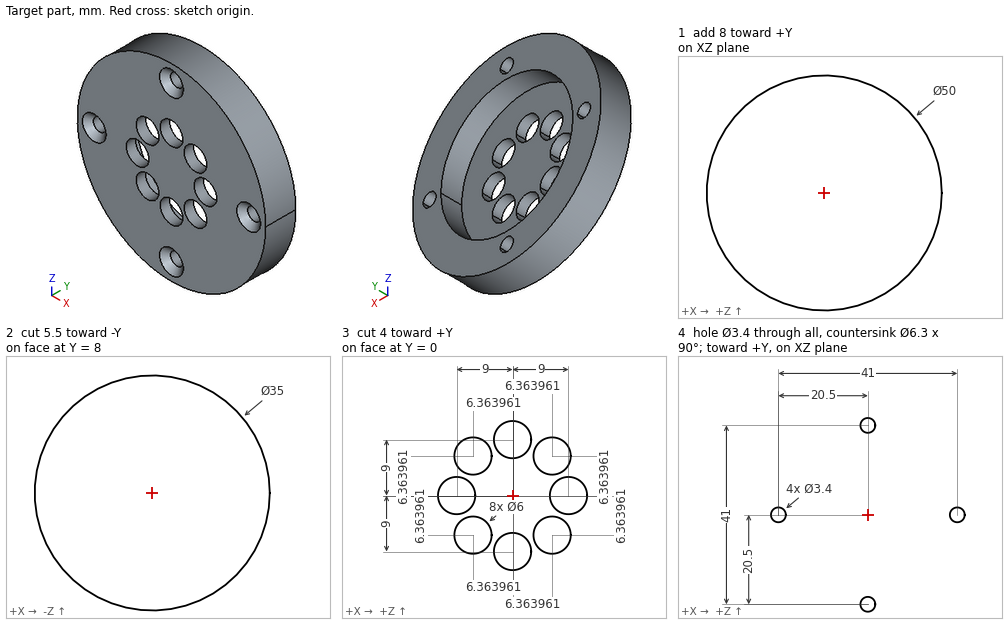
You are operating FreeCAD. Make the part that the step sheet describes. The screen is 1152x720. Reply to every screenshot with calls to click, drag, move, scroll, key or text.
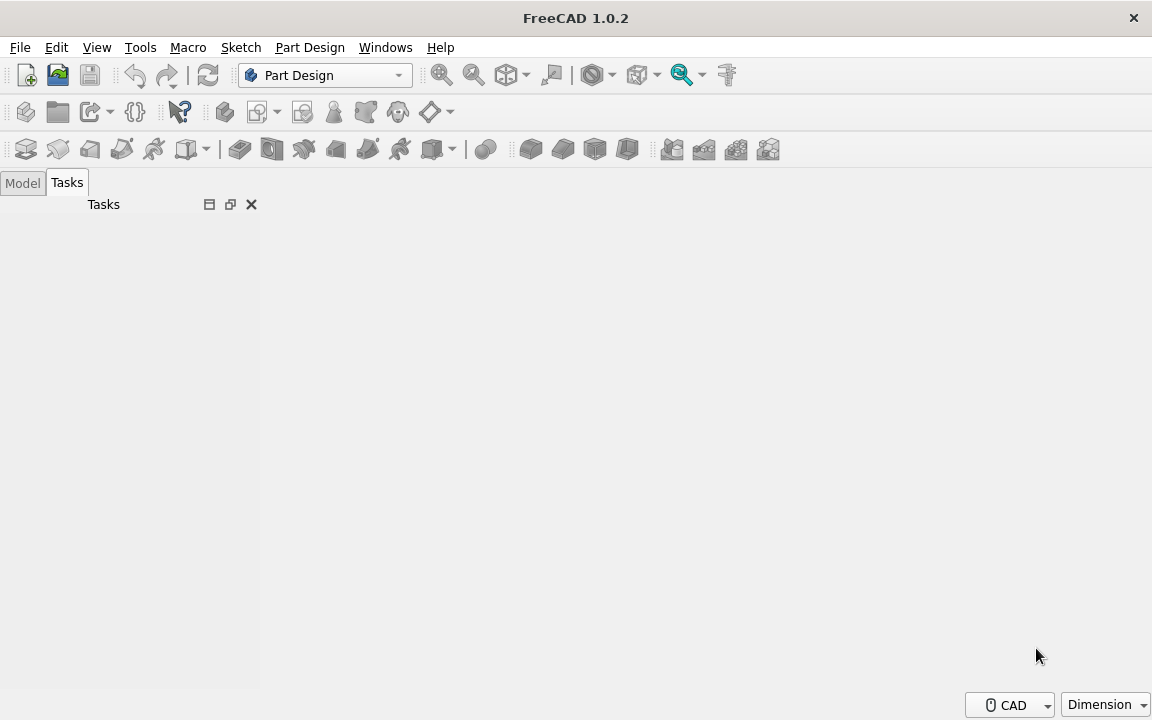
click(26, 76)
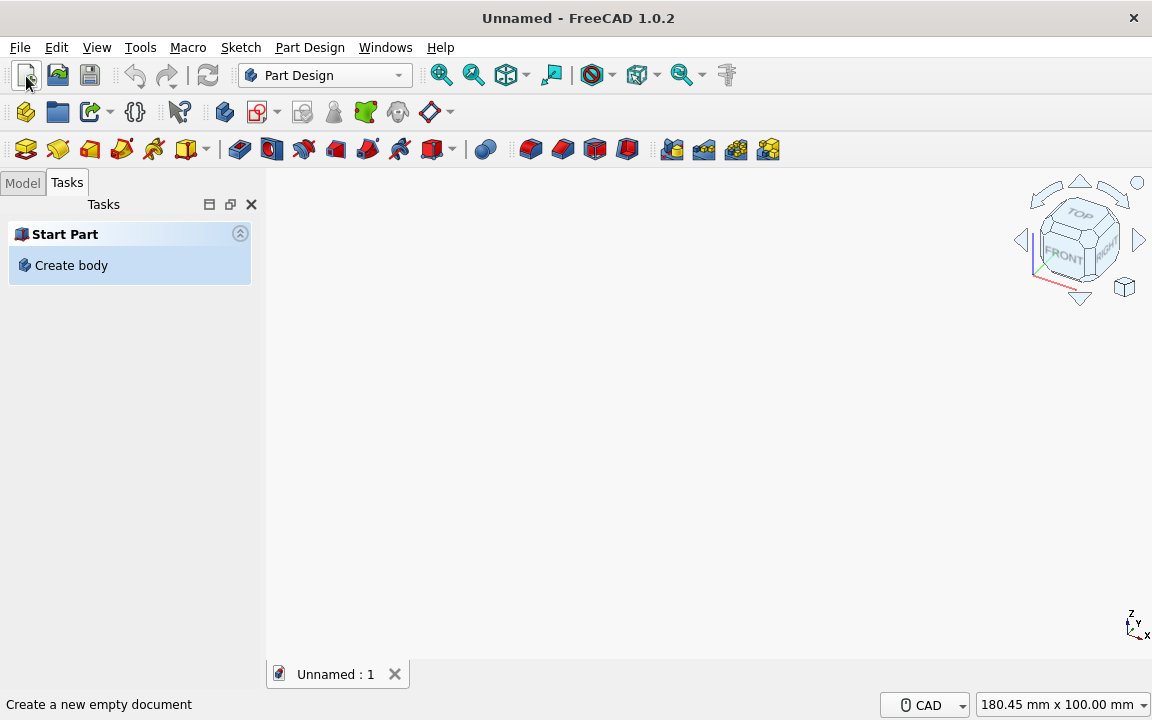
click(258, 112)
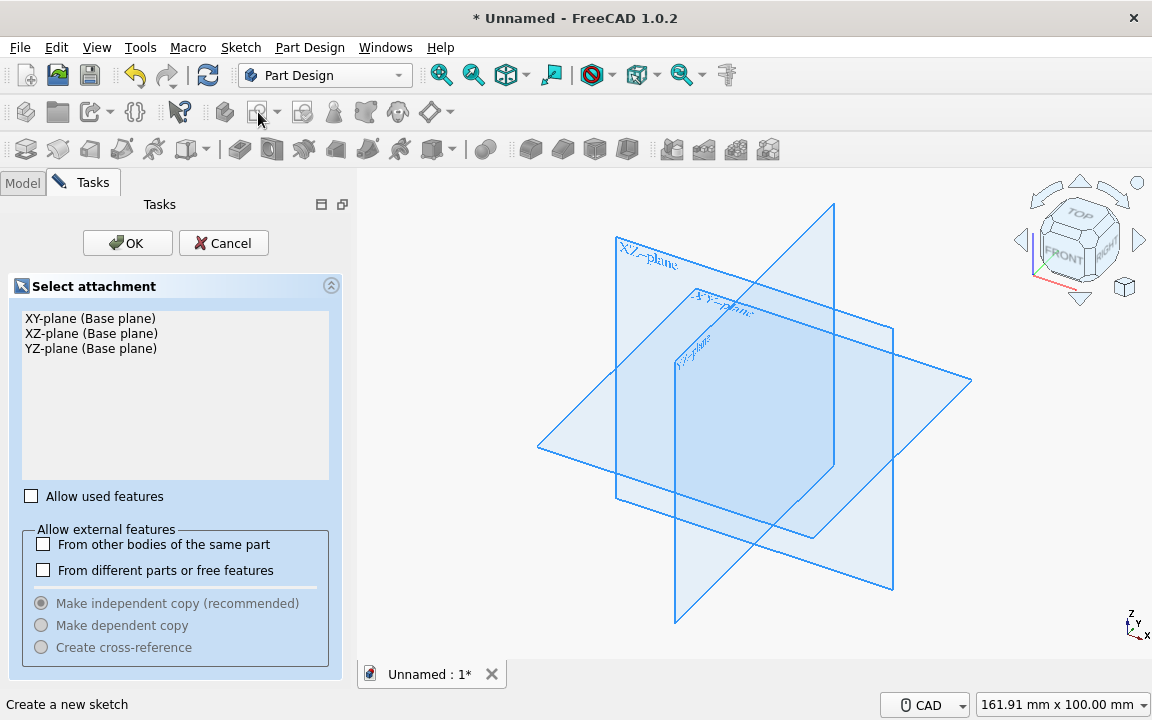
click(82, 334)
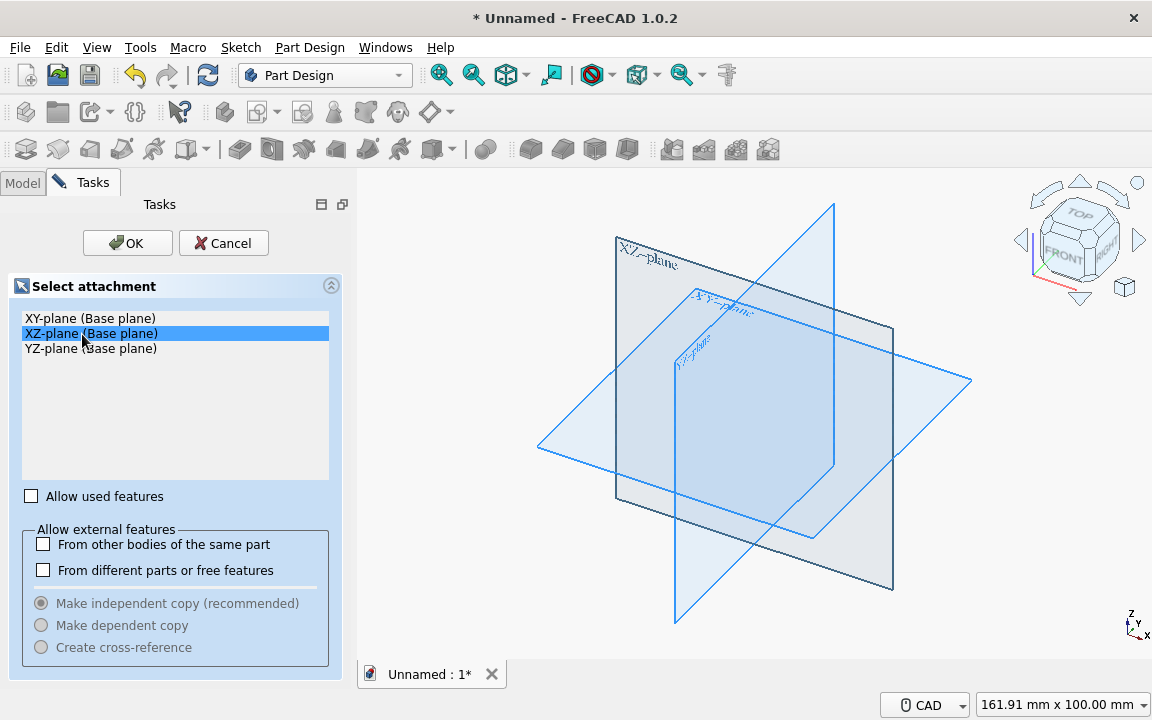
click(128, 243)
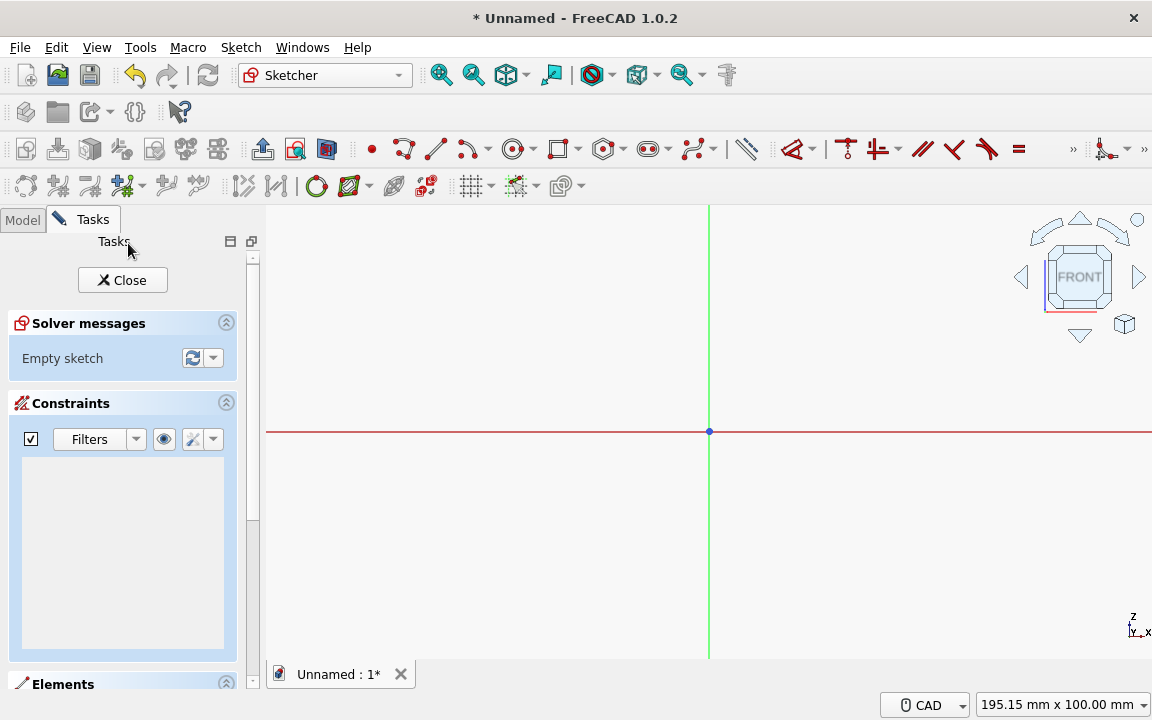
key(g)
key(c)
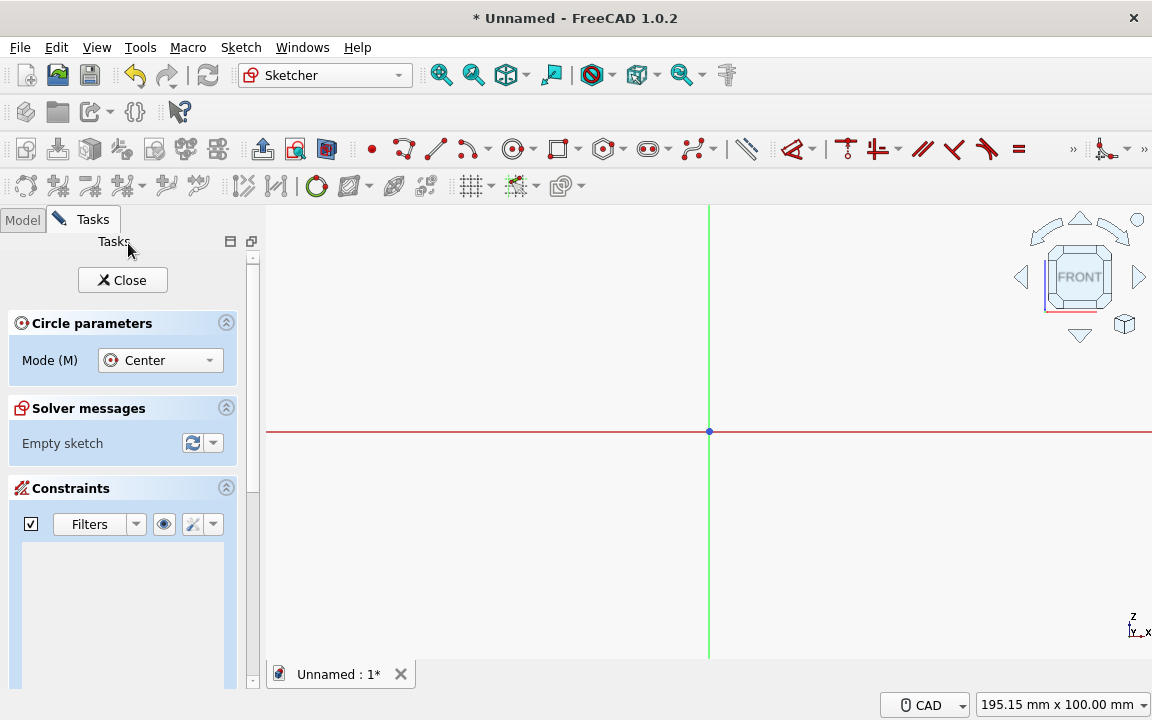
click(709, 432)
move(789, 352)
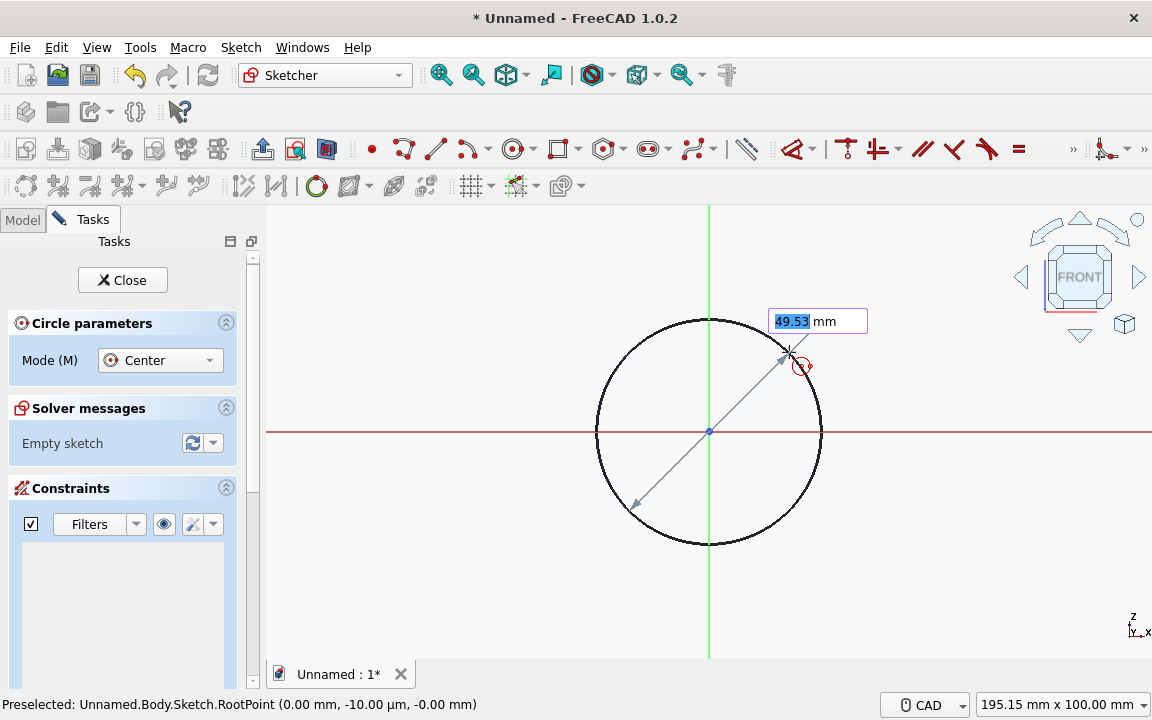
text(50)
key(Return)
key(Escape)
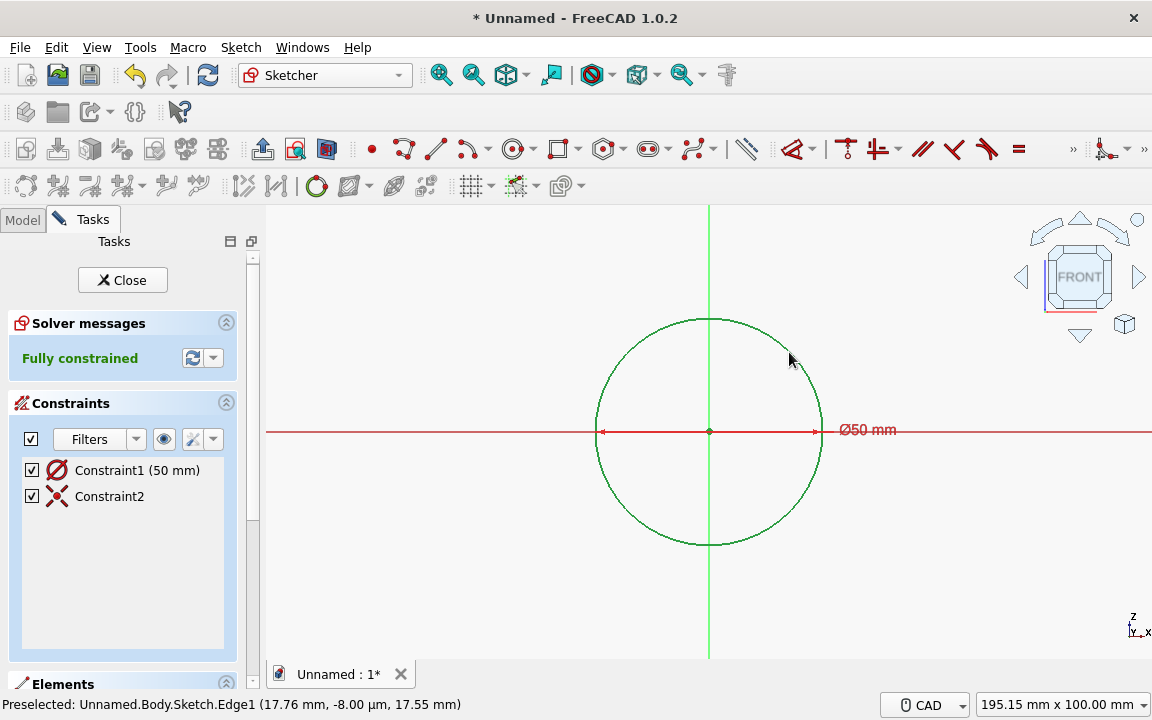
click(123, 280)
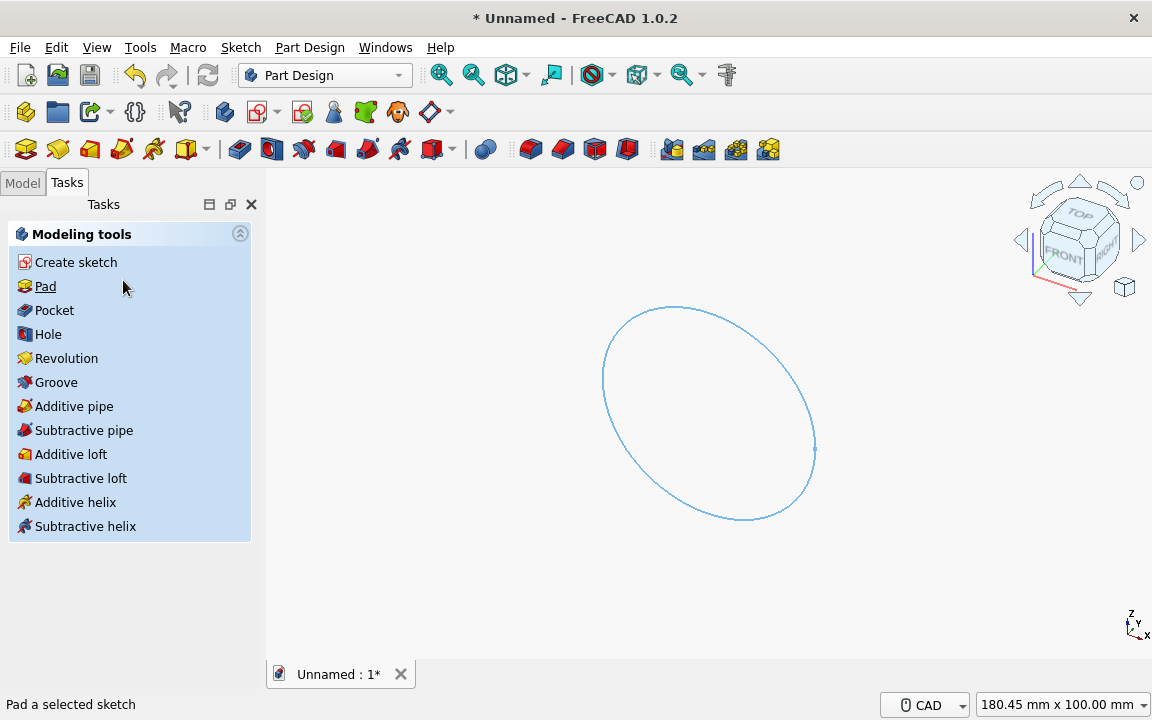
click(26, 150)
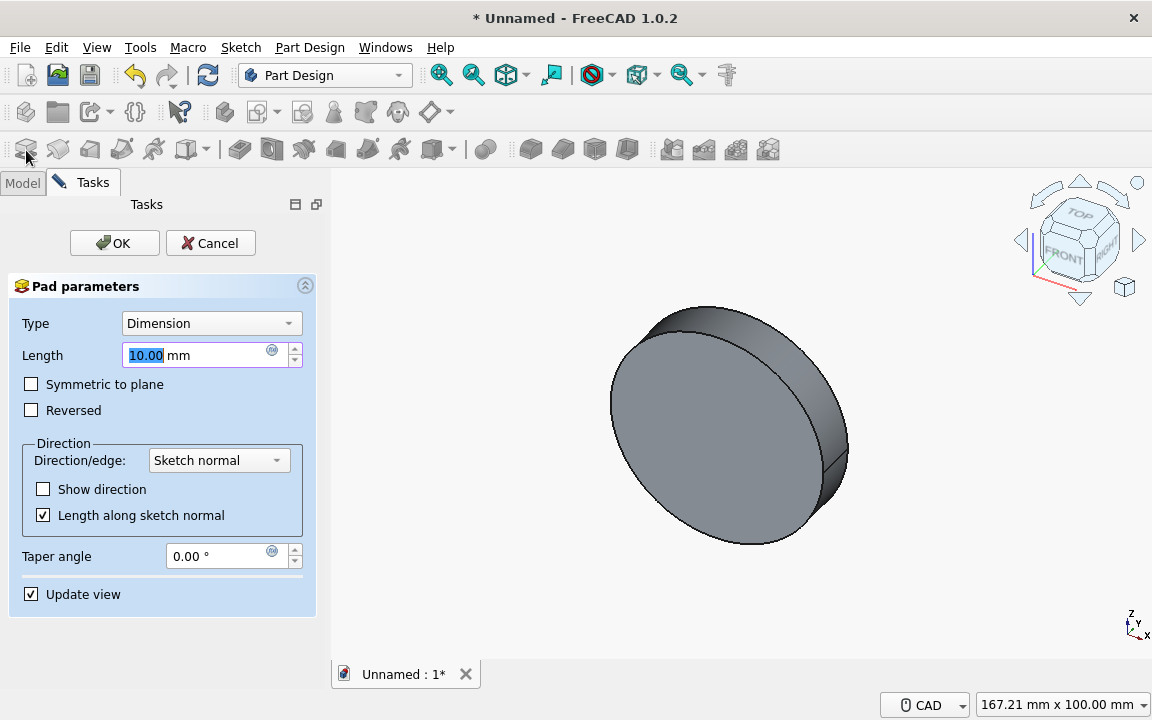
text(8)
key(Tab)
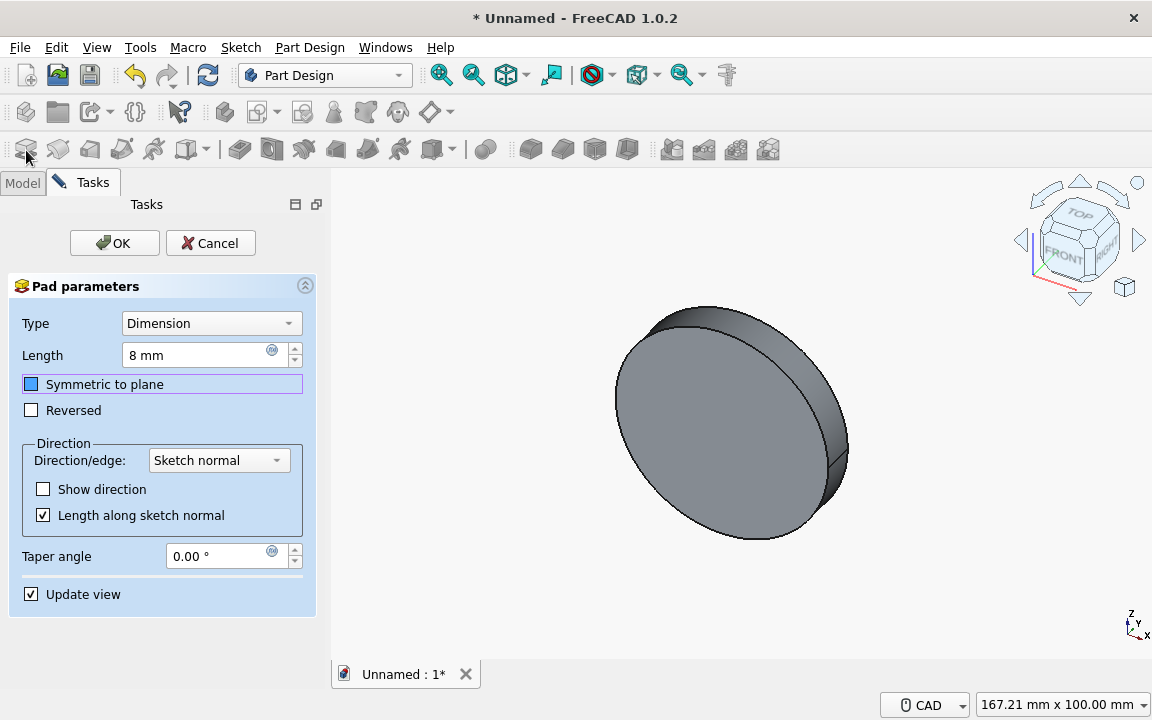
click(30, 410)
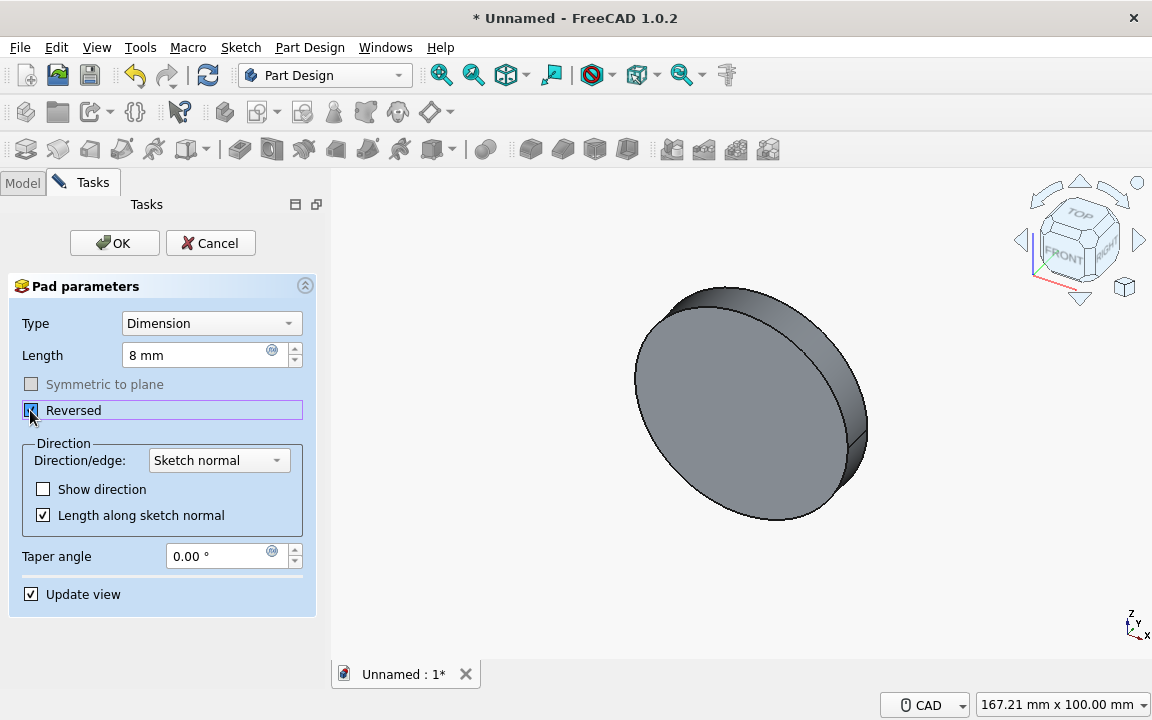
click(115, 243)